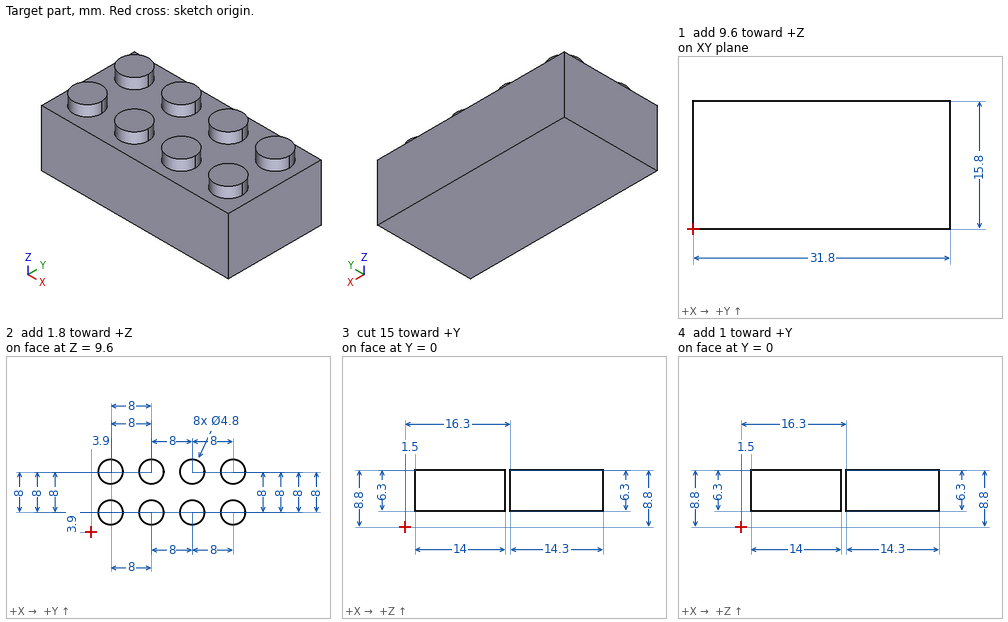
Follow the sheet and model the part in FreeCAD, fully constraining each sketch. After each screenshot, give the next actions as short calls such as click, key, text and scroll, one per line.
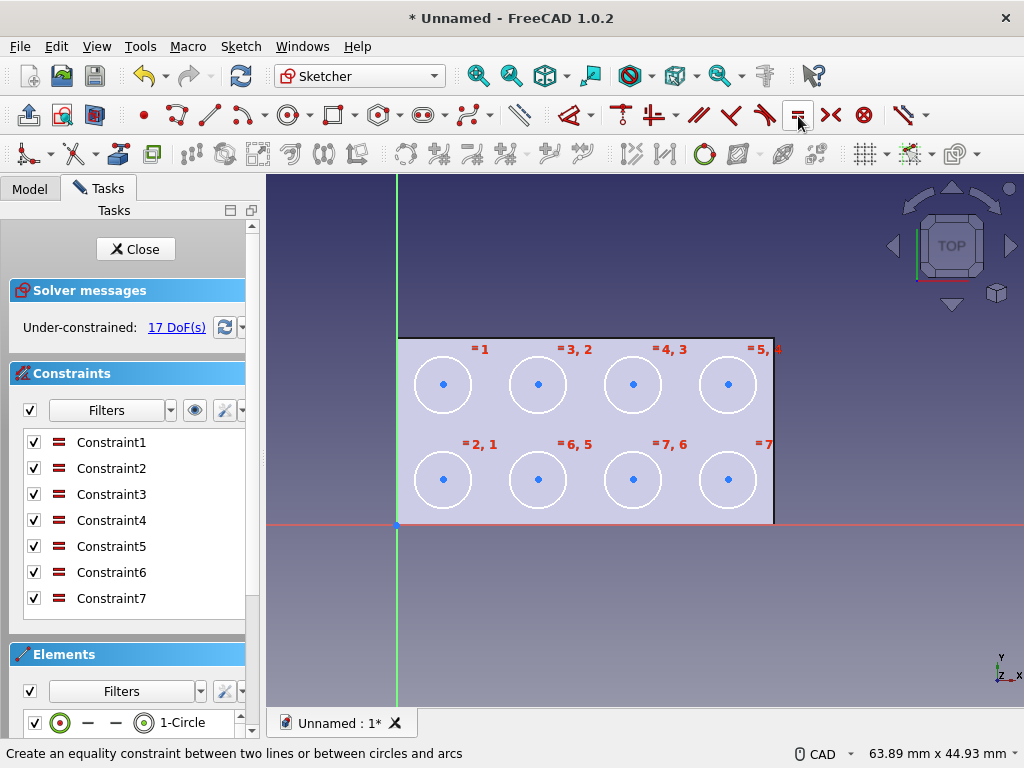
click(463, 365)
click(486, 342)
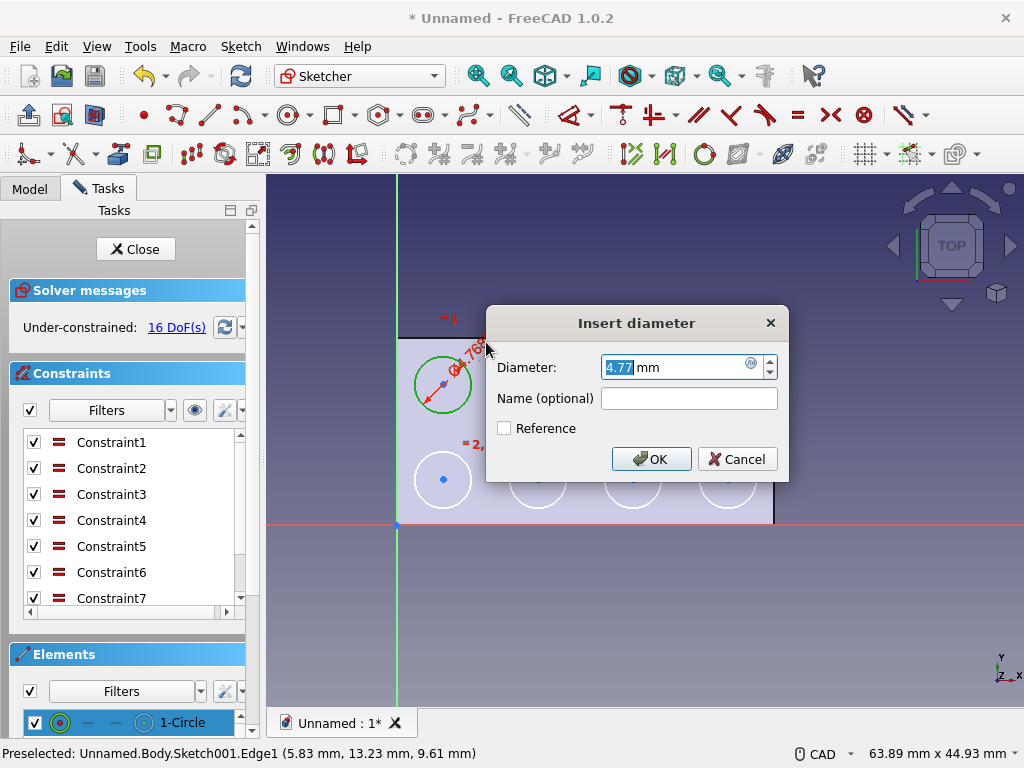
text(4.8)
key(Return)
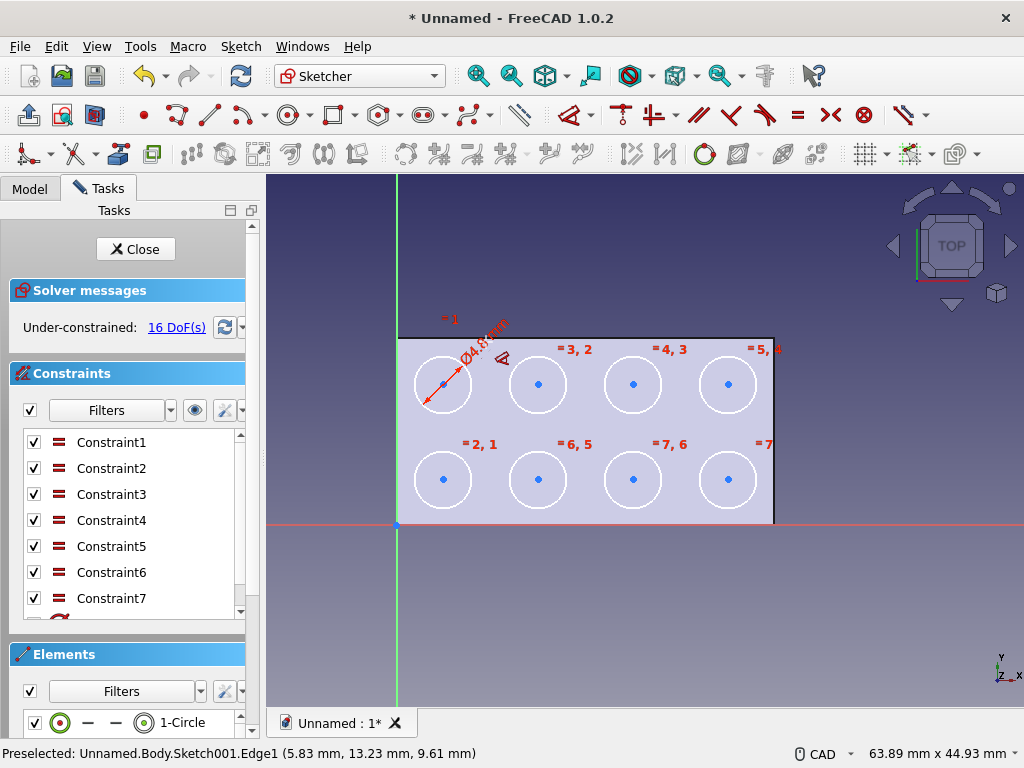
click(443, 385)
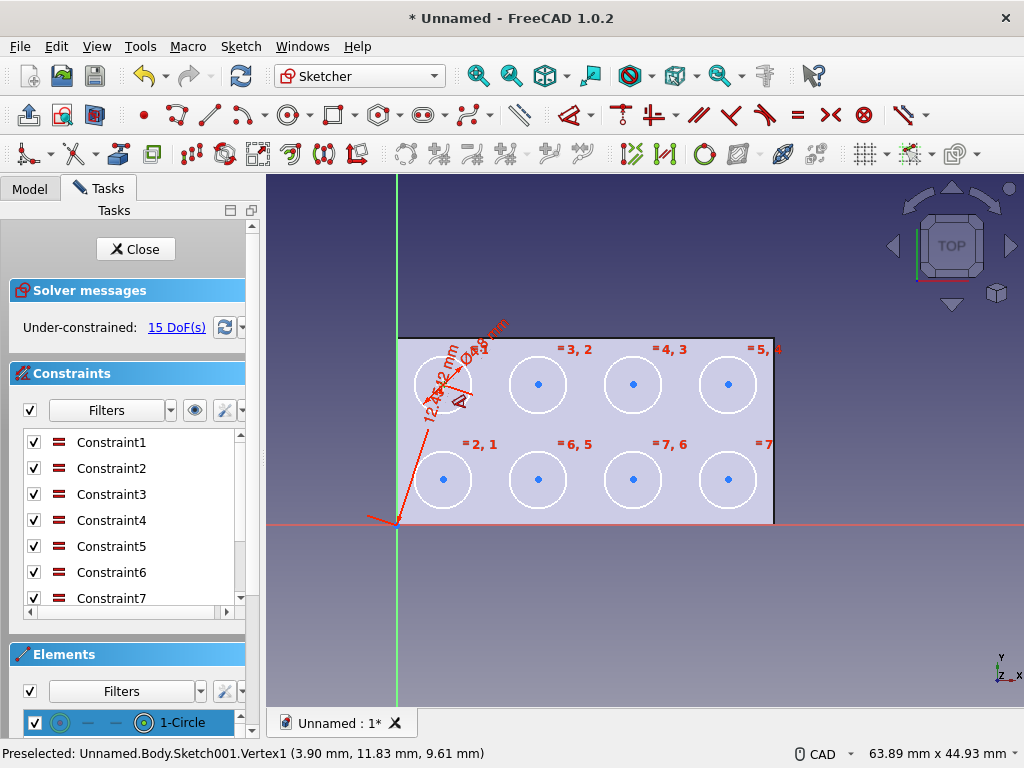
click(443, 480)
click(477, 432)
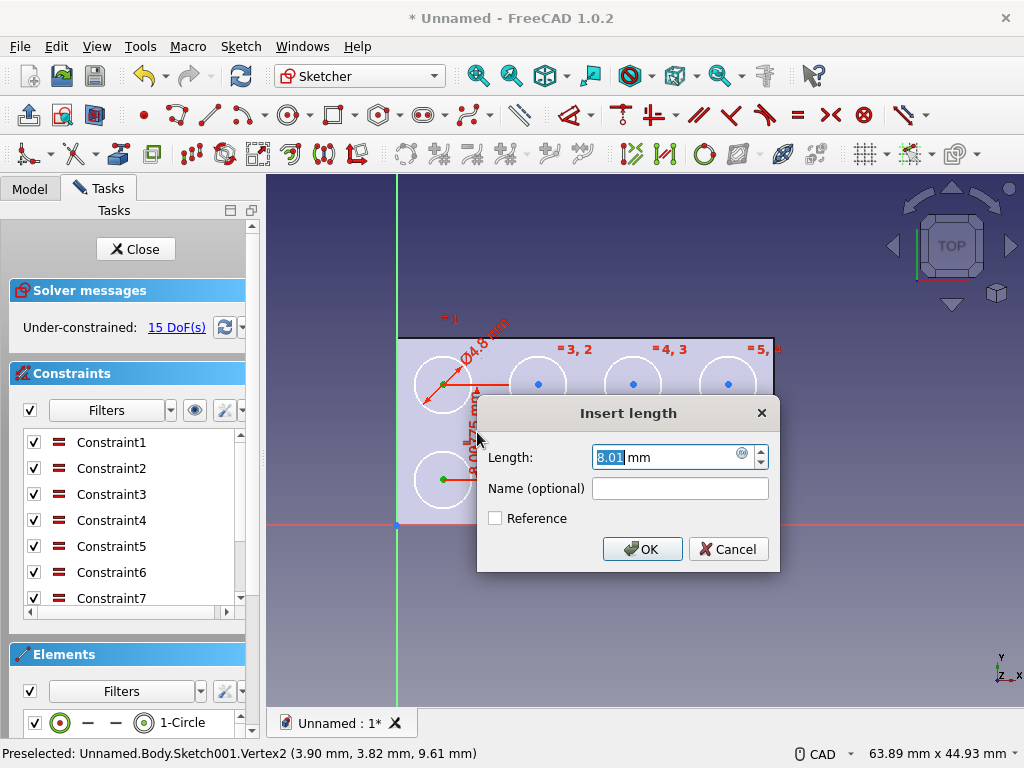
text(8)
key(Return)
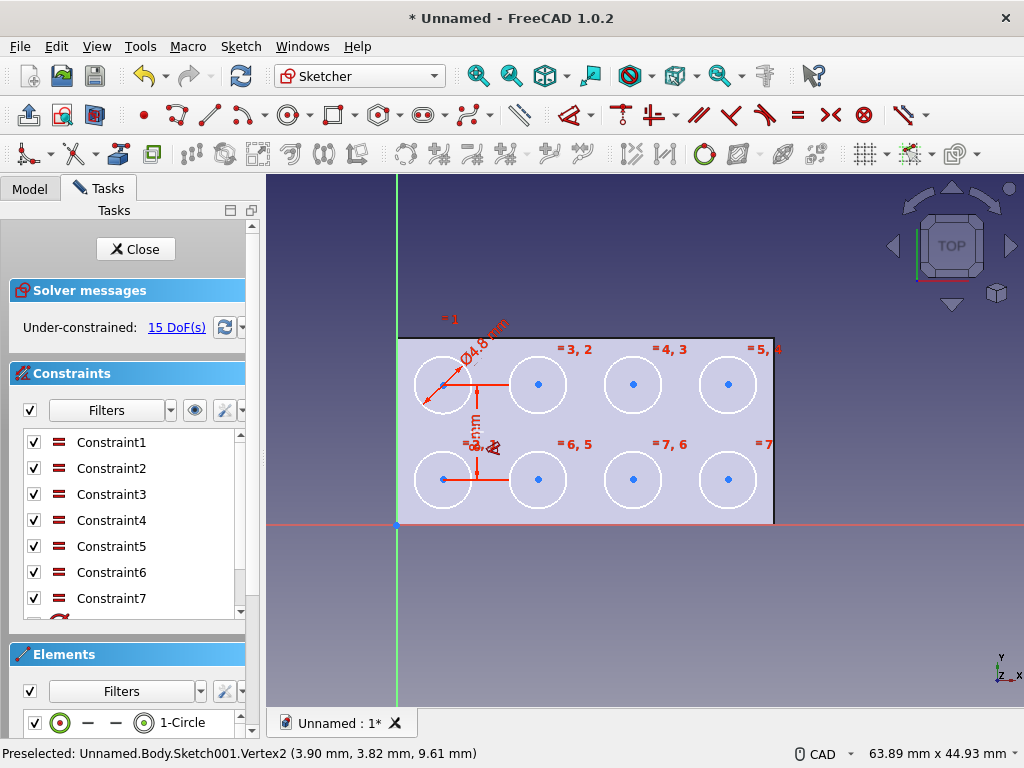
click(443, 385)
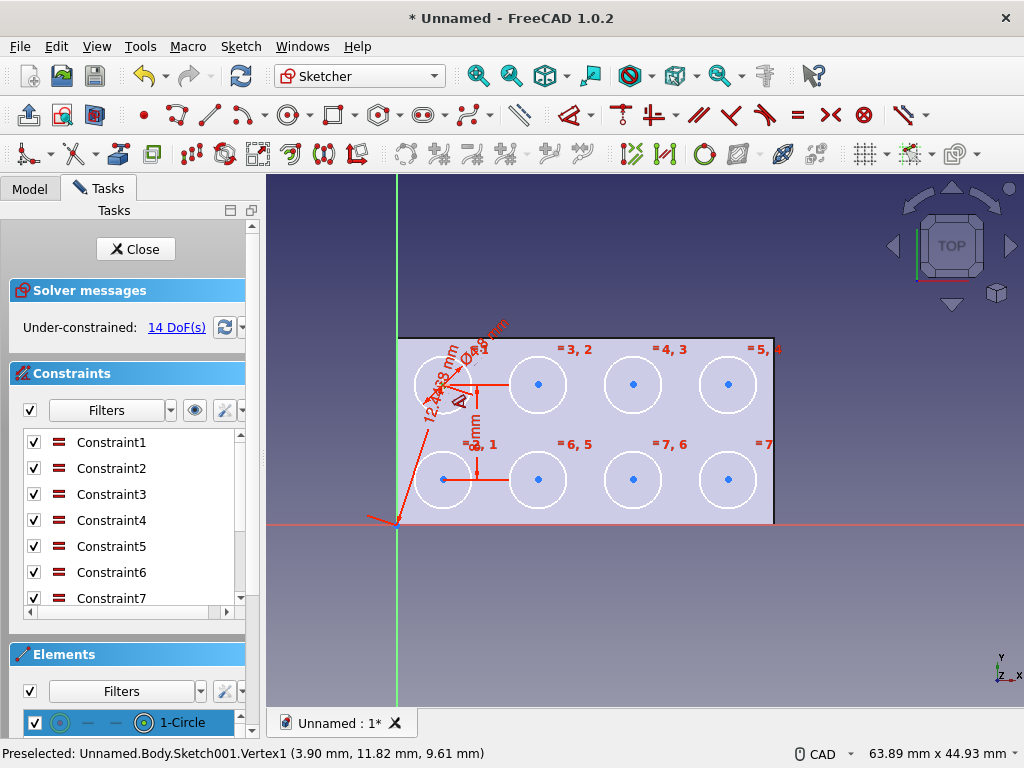
click(538, 385)
click(491, 303)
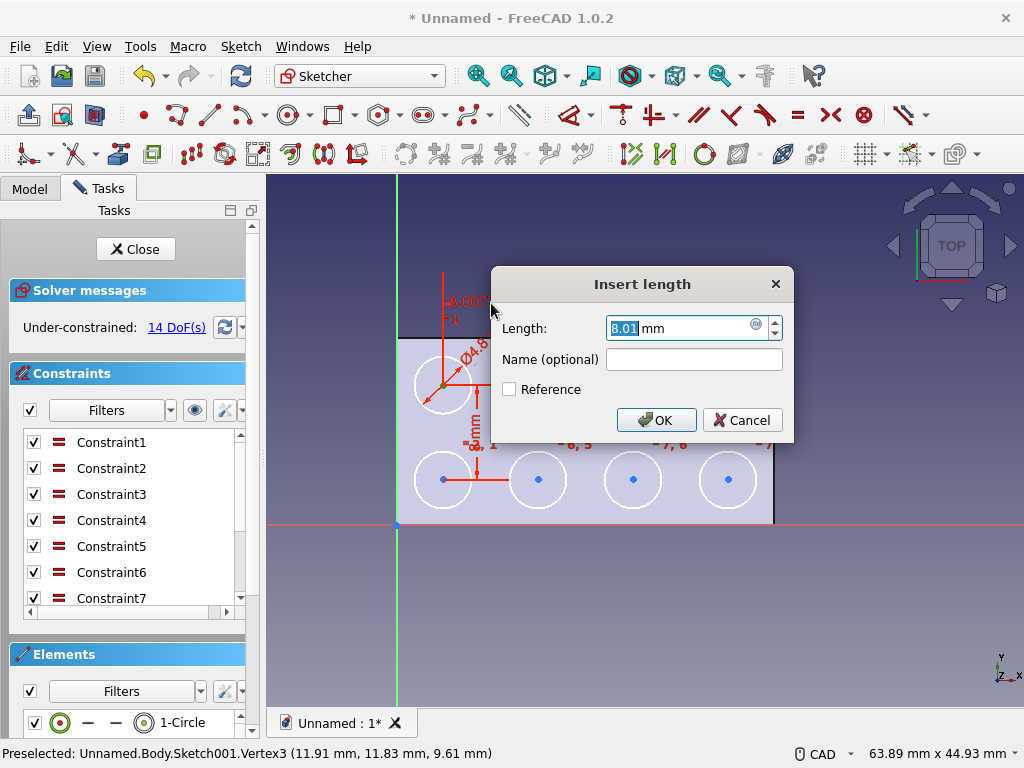
text(8)
key(Return)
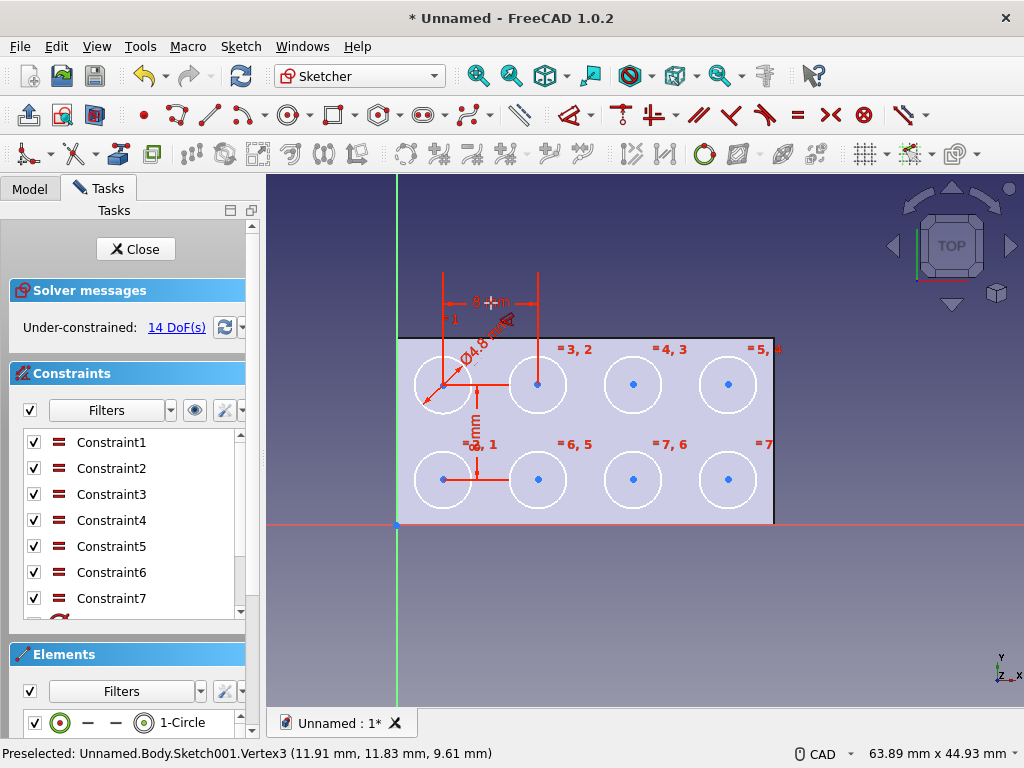
click(443, 480)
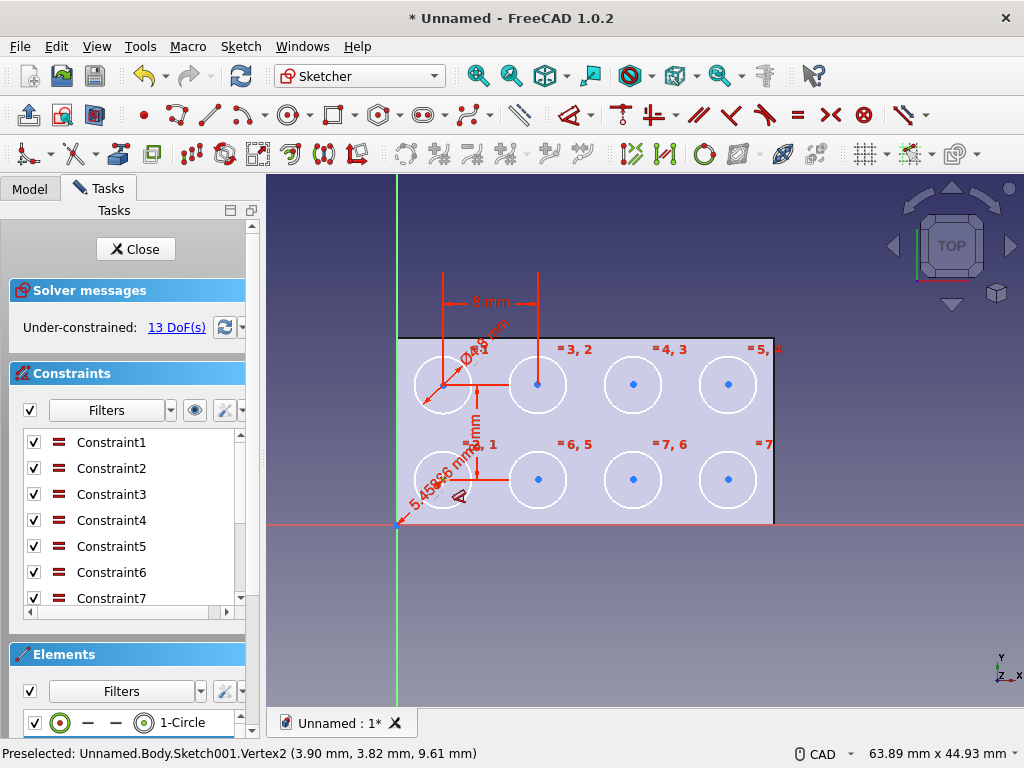
click(538, 385)
click(490, 562)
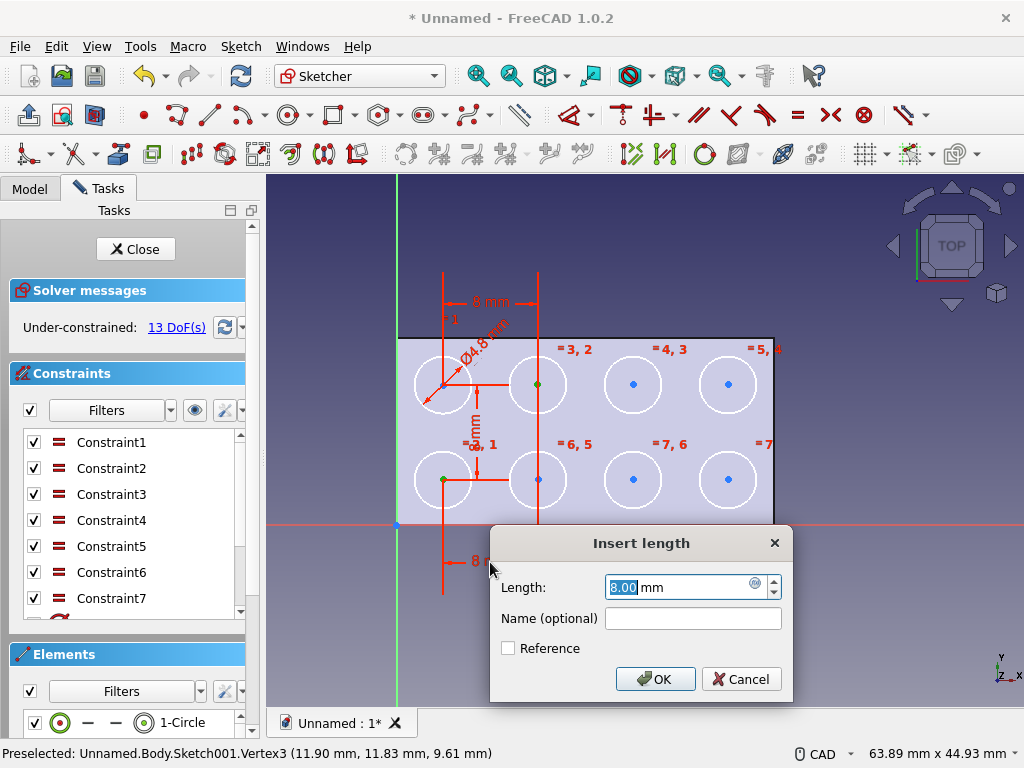
text(8)
key(Return)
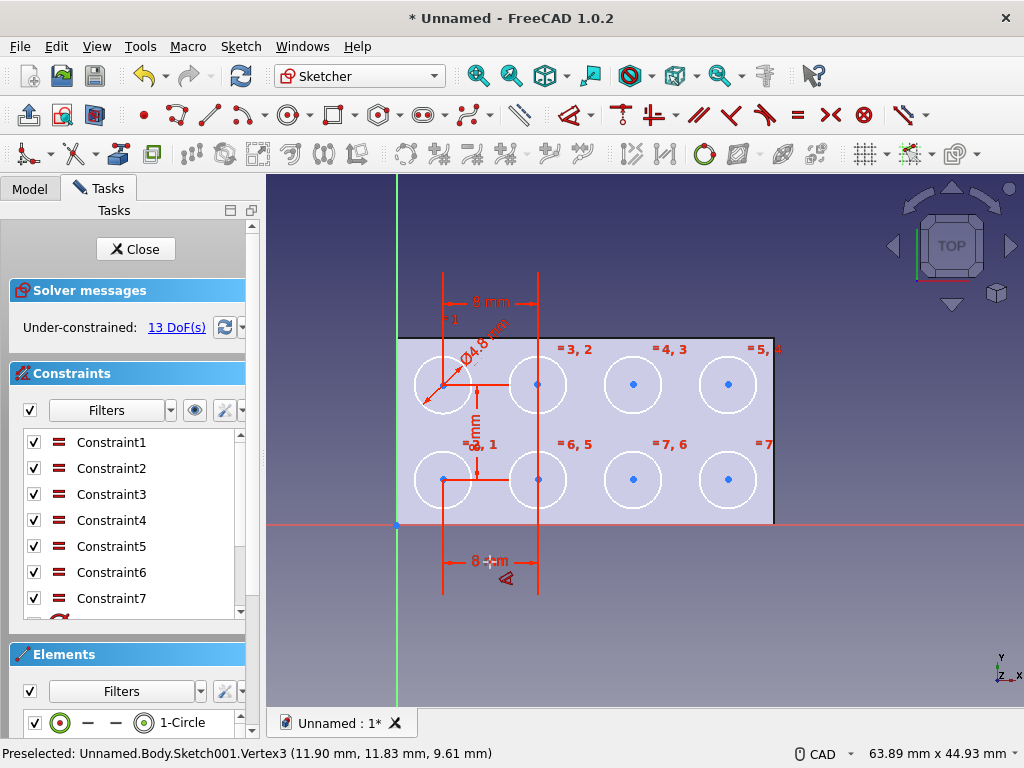
click(443, 480)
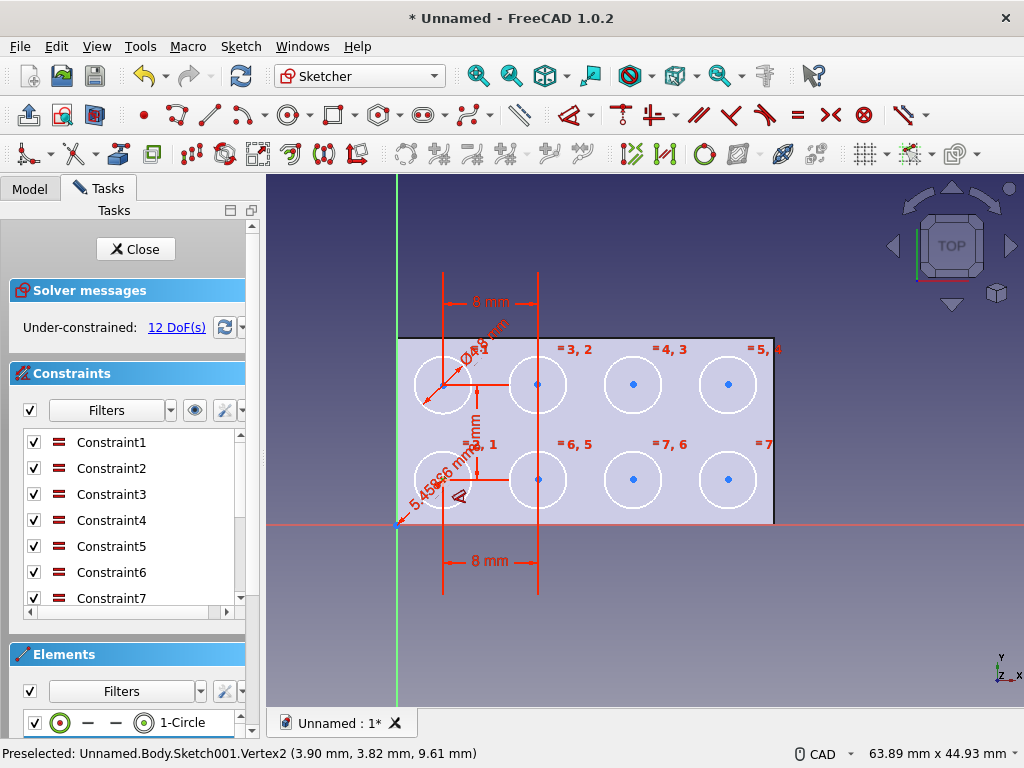
click(538, 385)
click(572, 432)